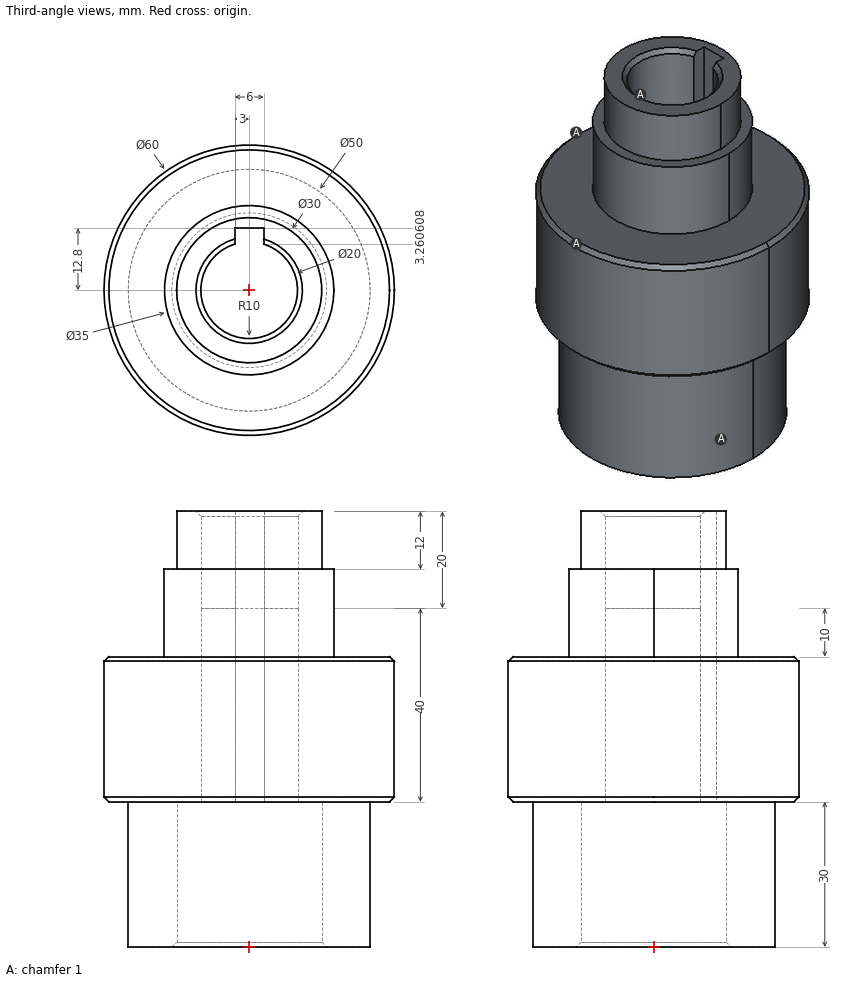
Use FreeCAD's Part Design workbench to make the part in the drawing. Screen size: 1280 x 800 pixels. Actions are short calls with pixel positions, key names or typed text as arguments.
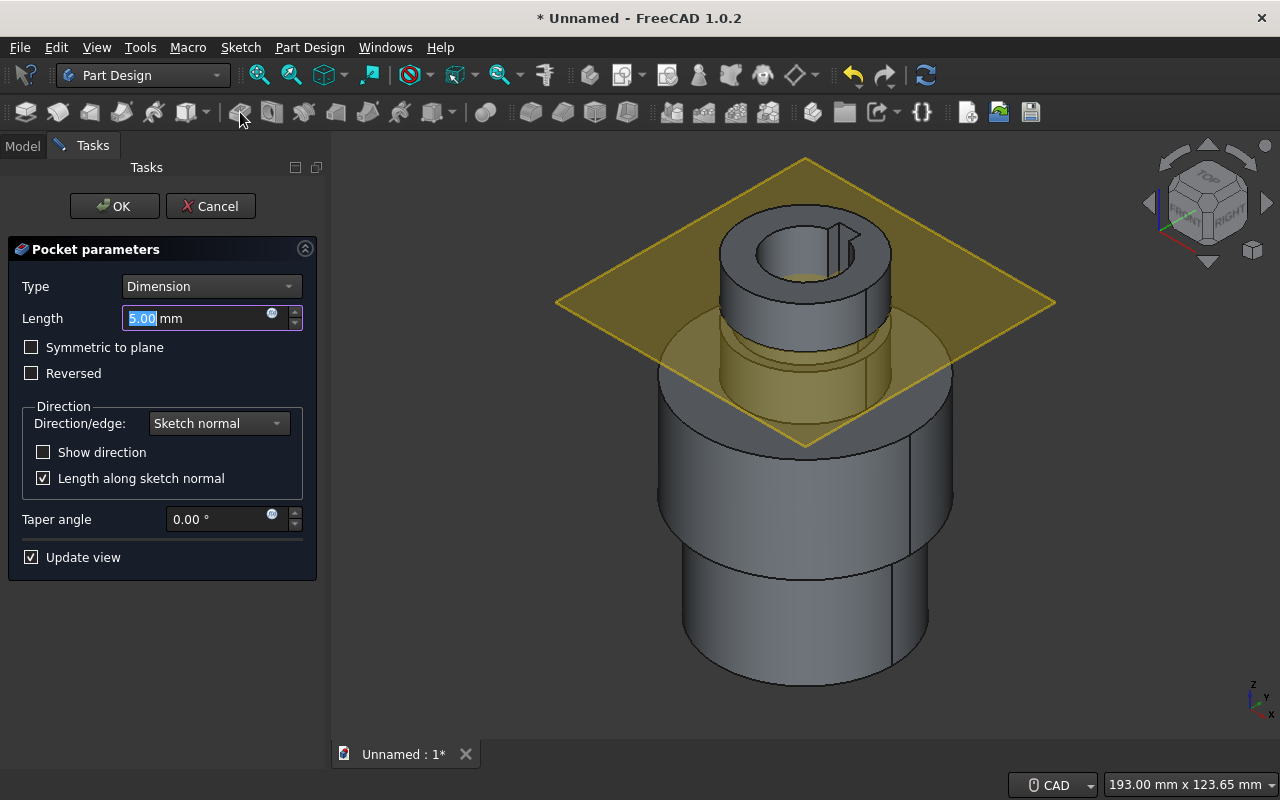
text(12)
key(Tab)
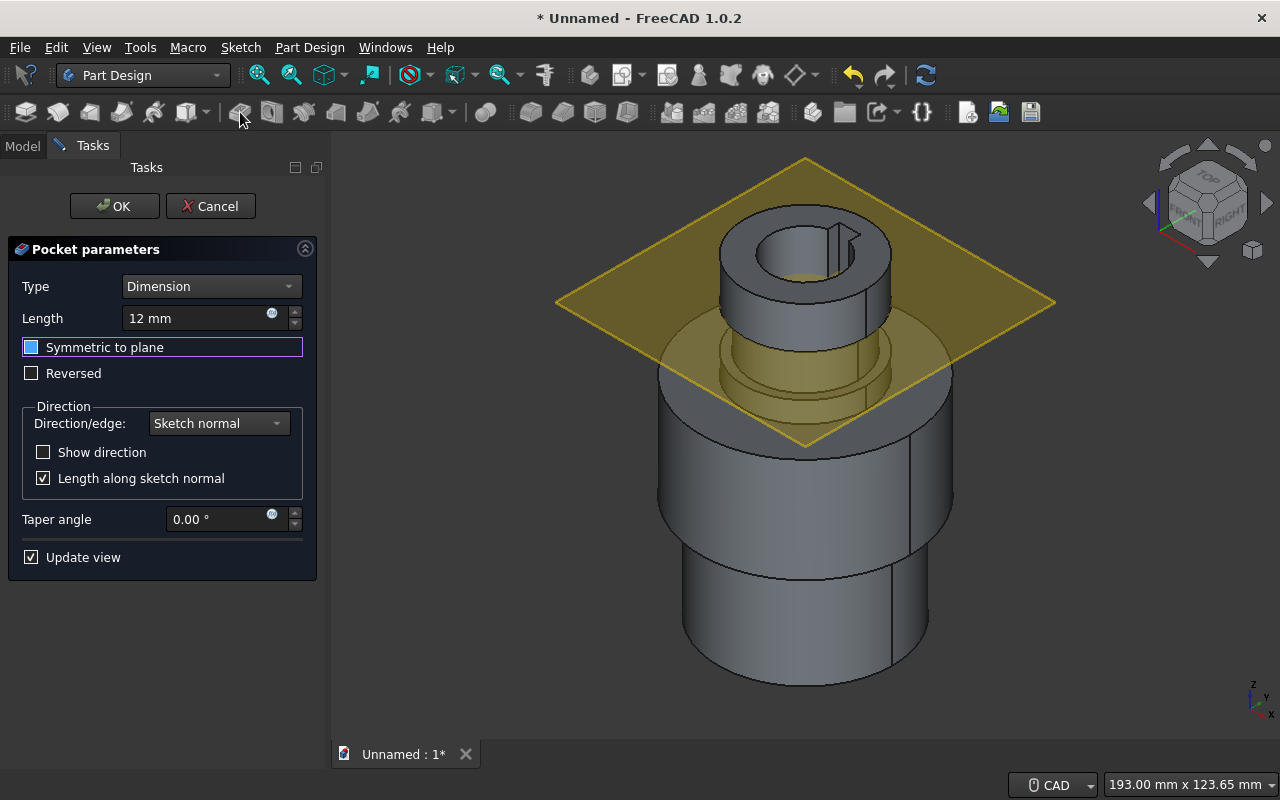
click(30, 373)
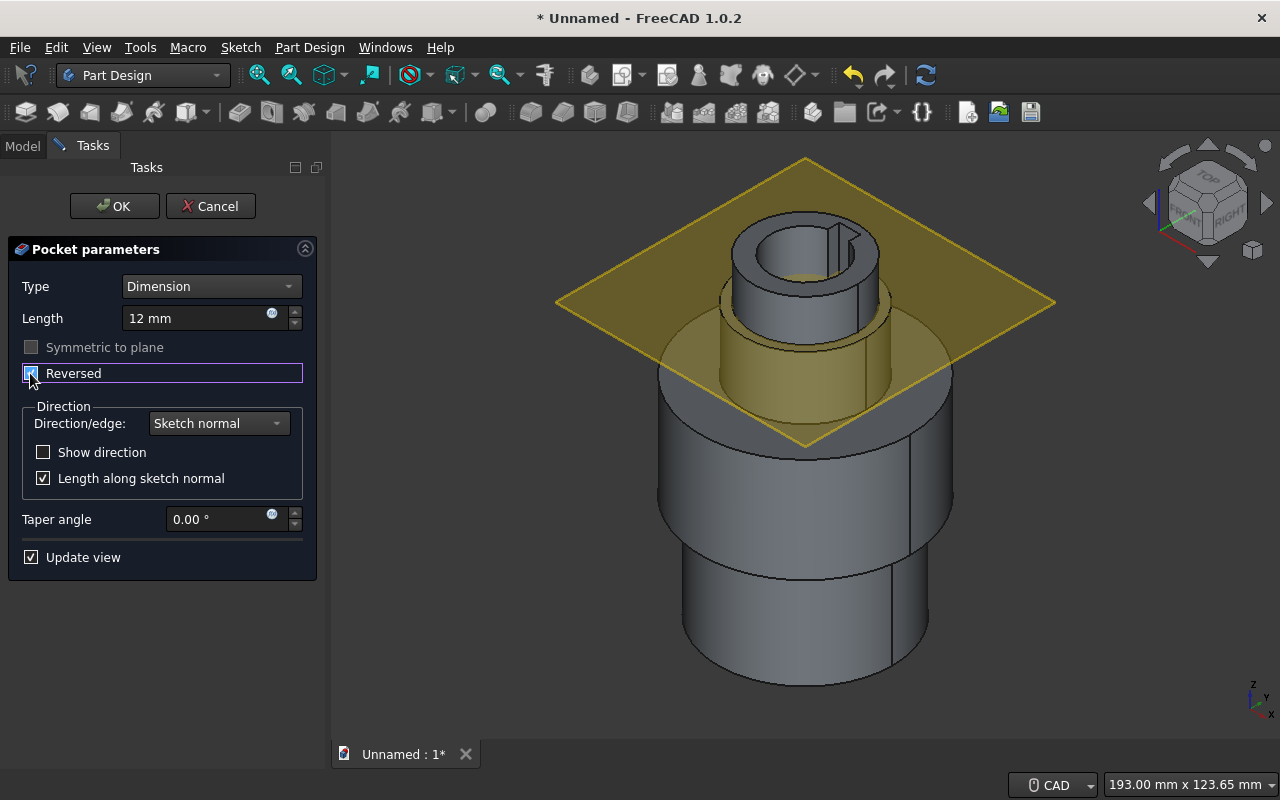
click(115, 206)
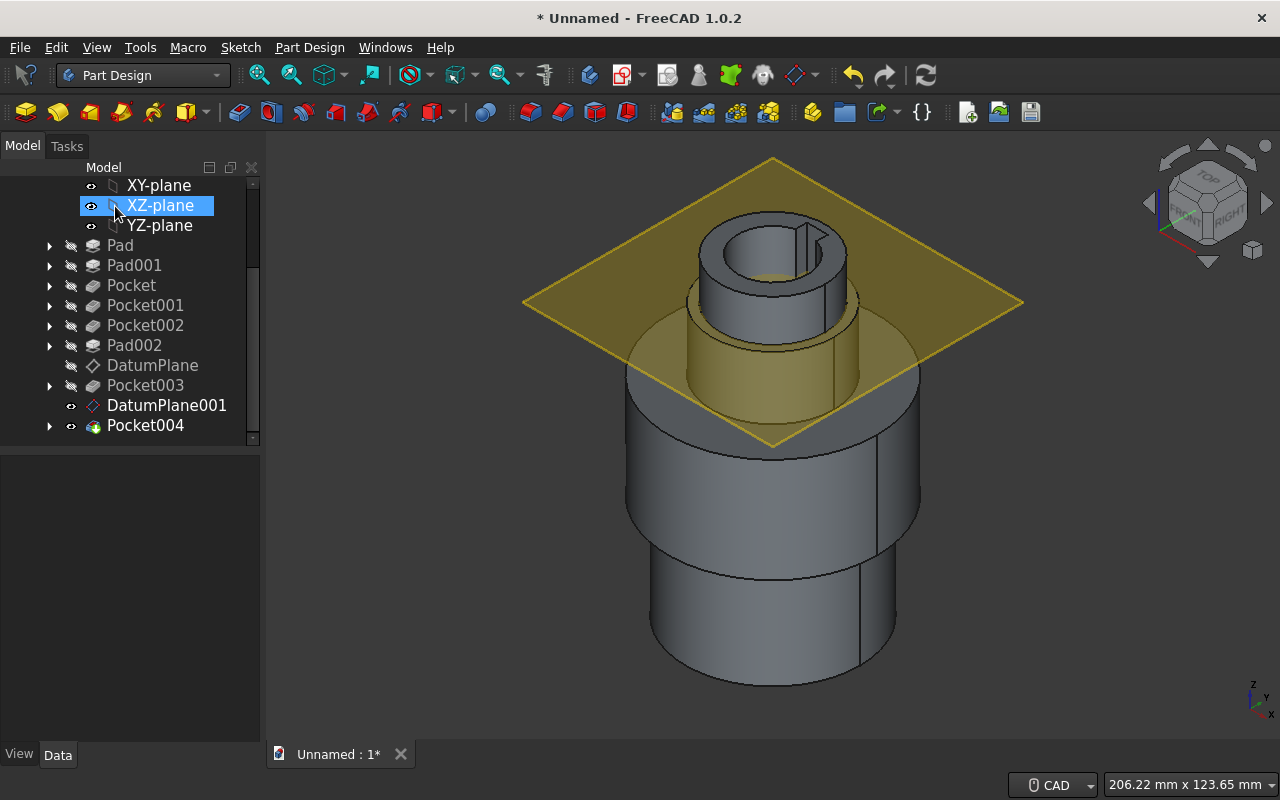
click(116, 406)
key(space)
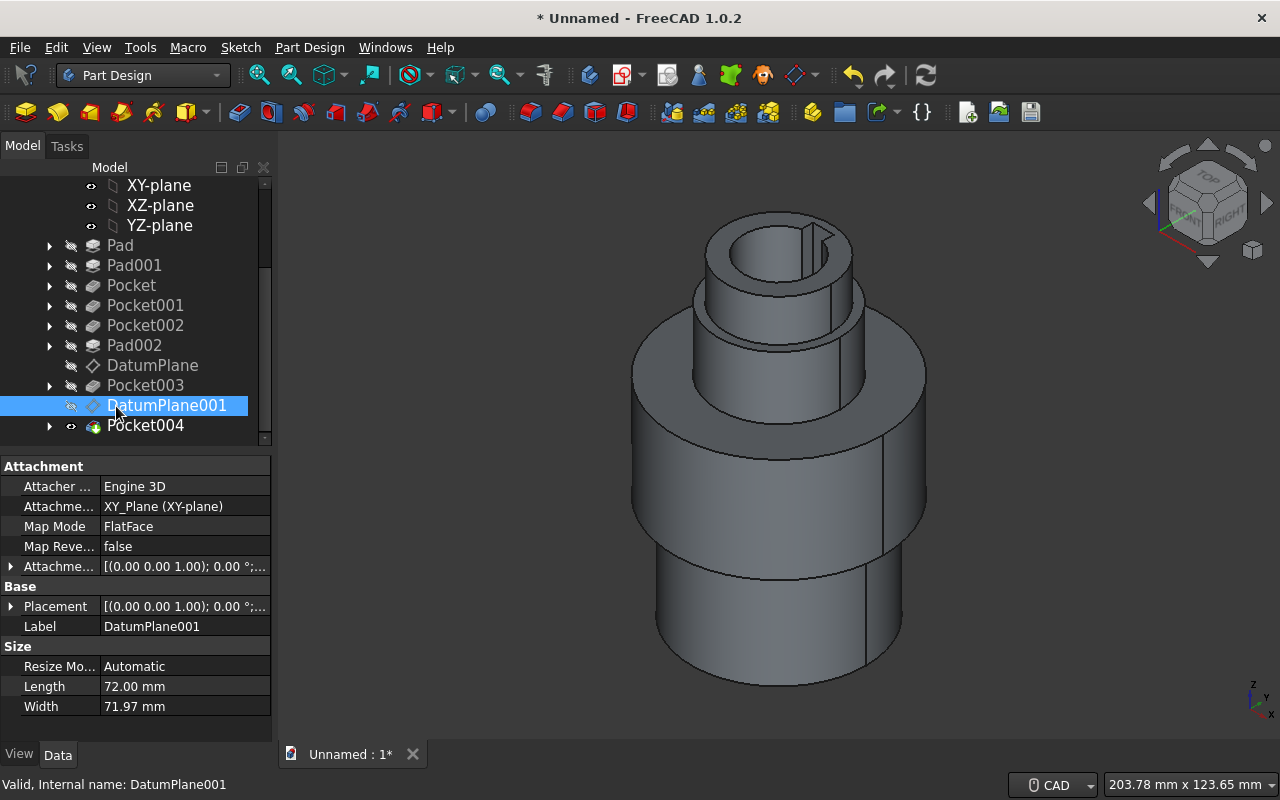
click(733, 244)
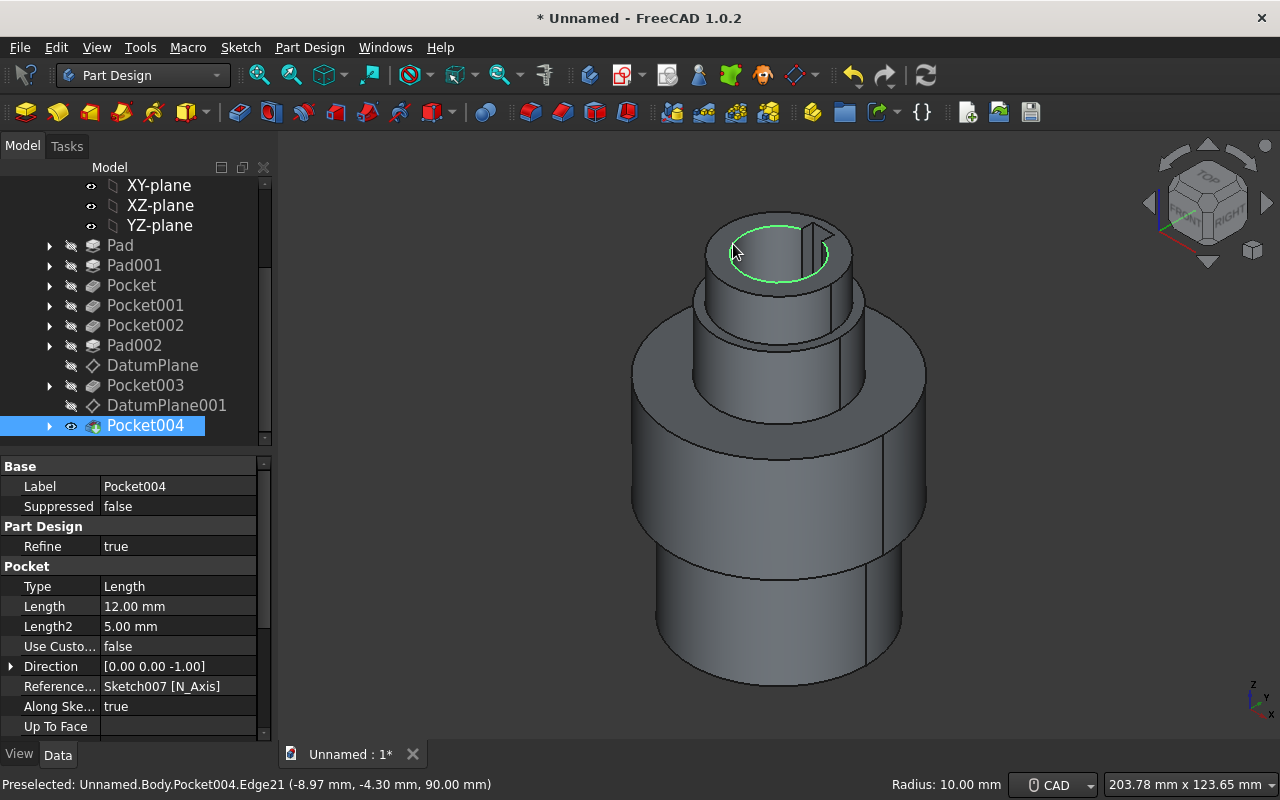
click(647, 412, ctrl)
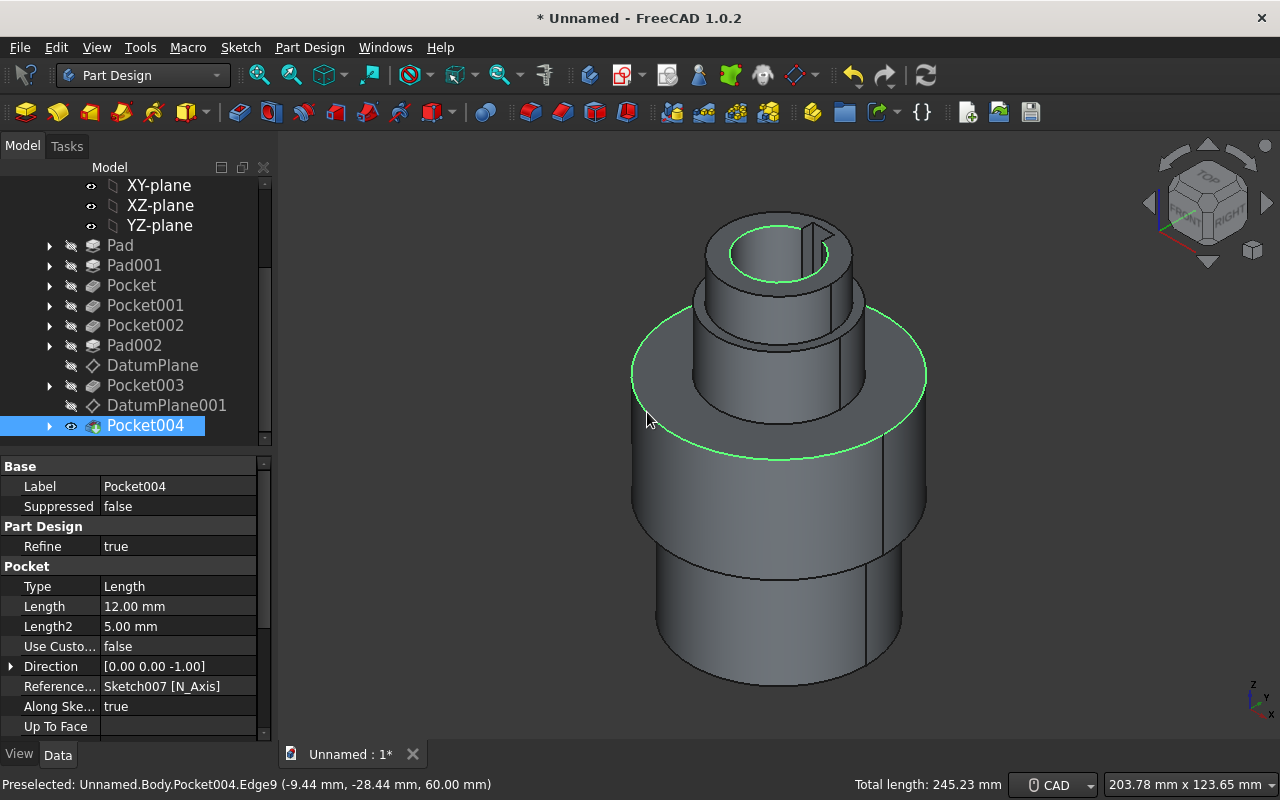
key(2)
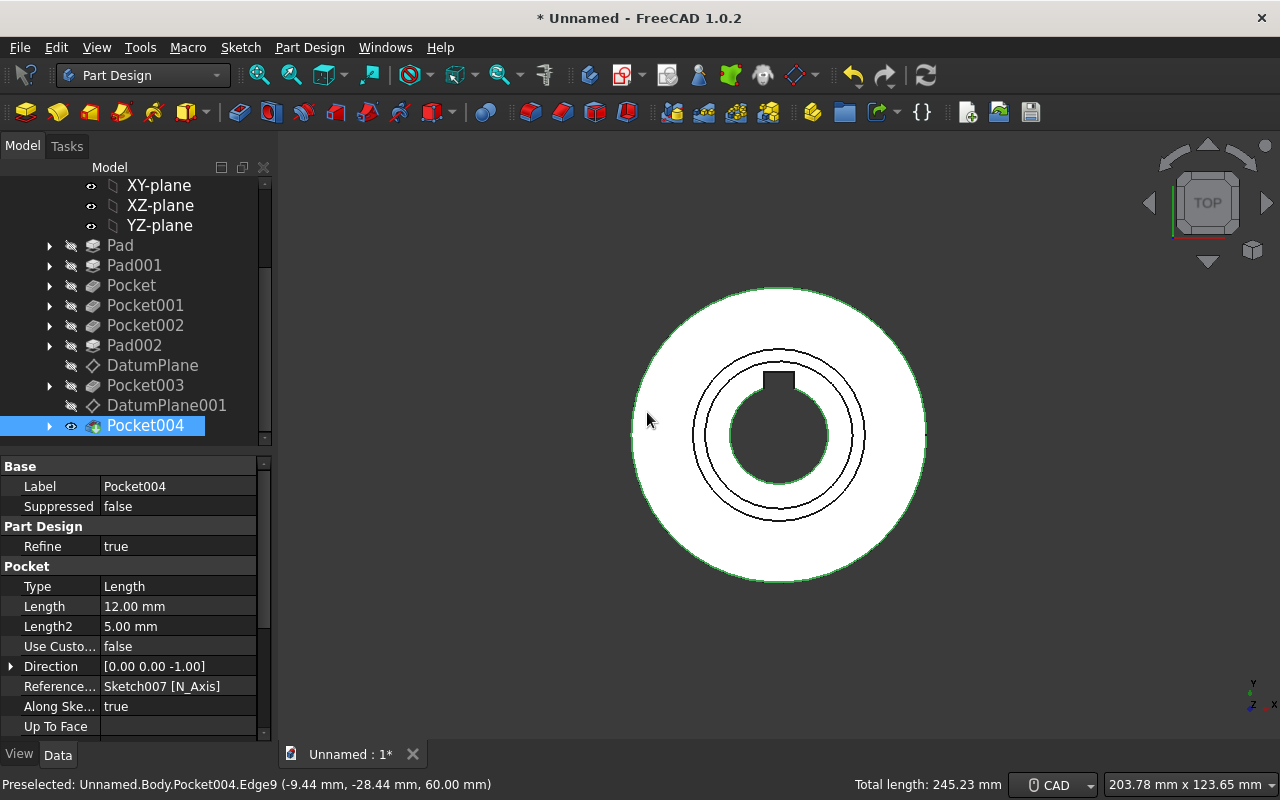
key(0)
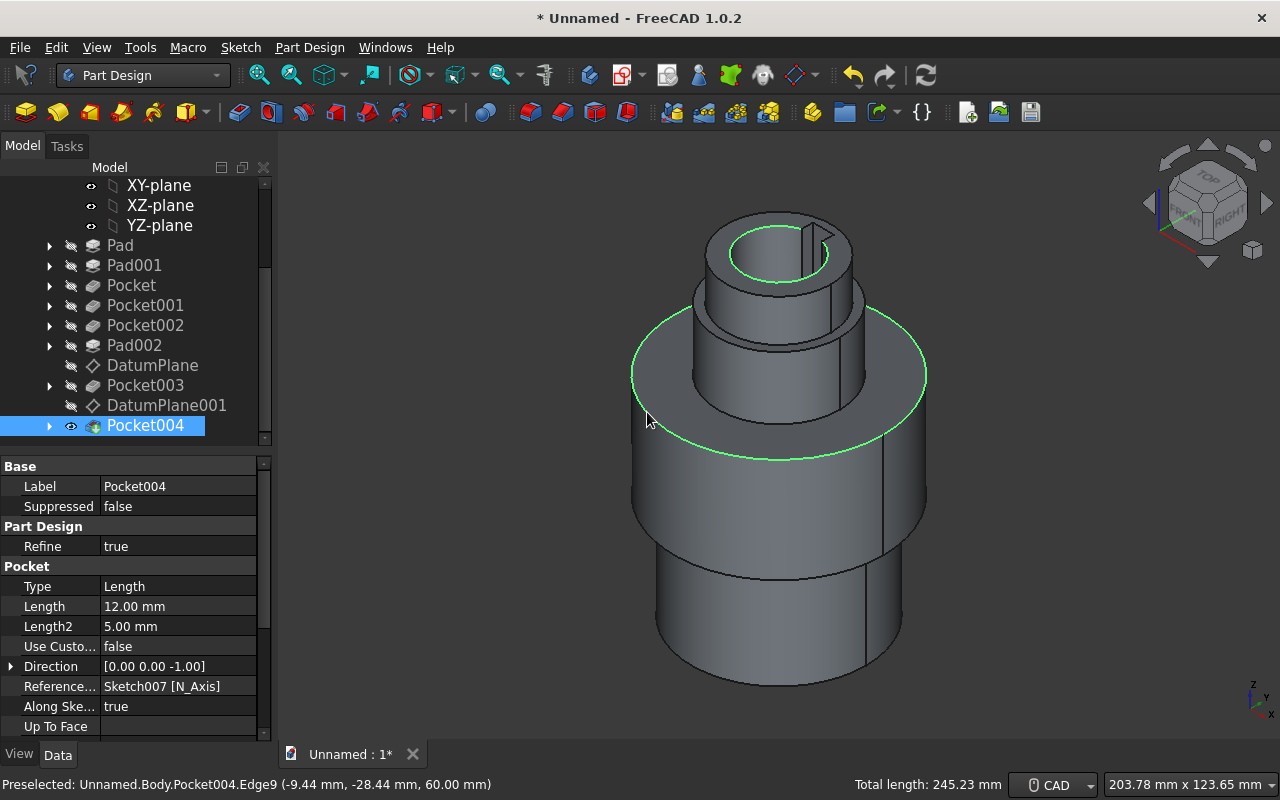
key(1)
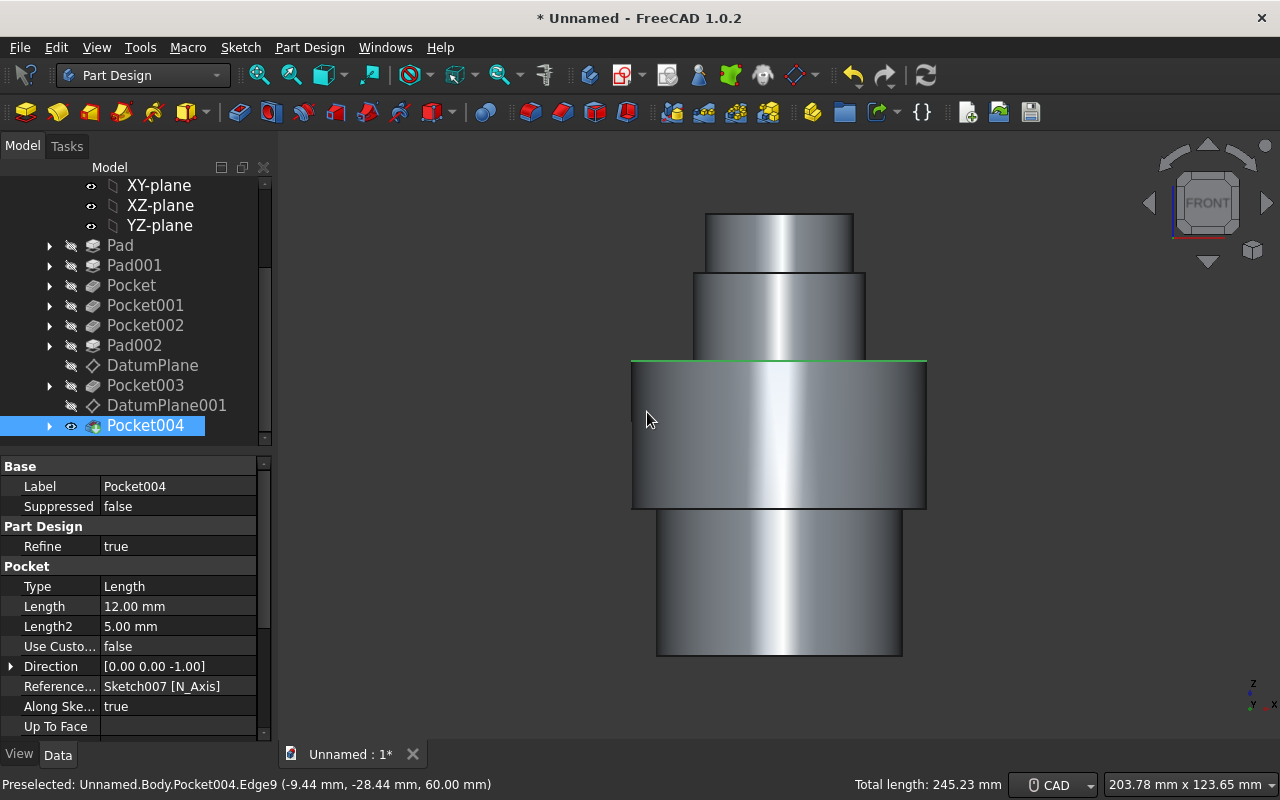
click(824, 508, ctrl)